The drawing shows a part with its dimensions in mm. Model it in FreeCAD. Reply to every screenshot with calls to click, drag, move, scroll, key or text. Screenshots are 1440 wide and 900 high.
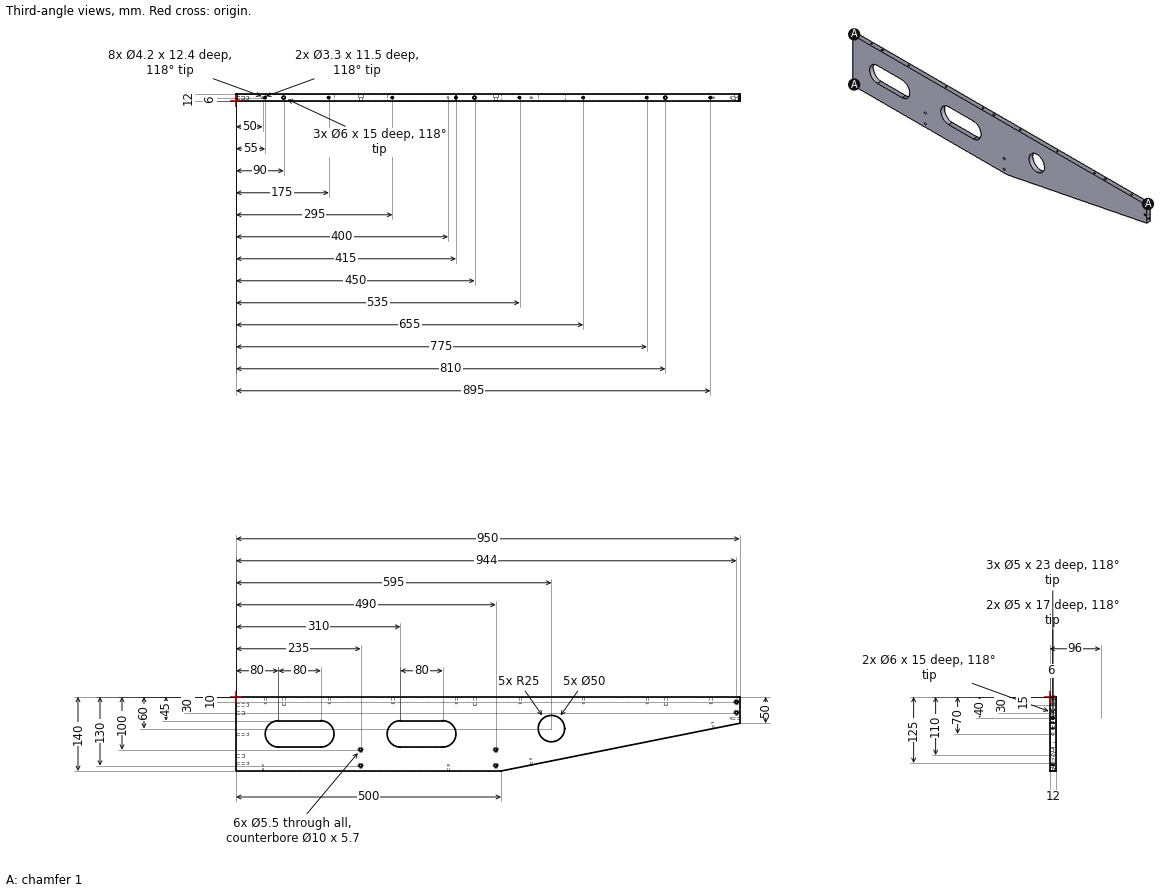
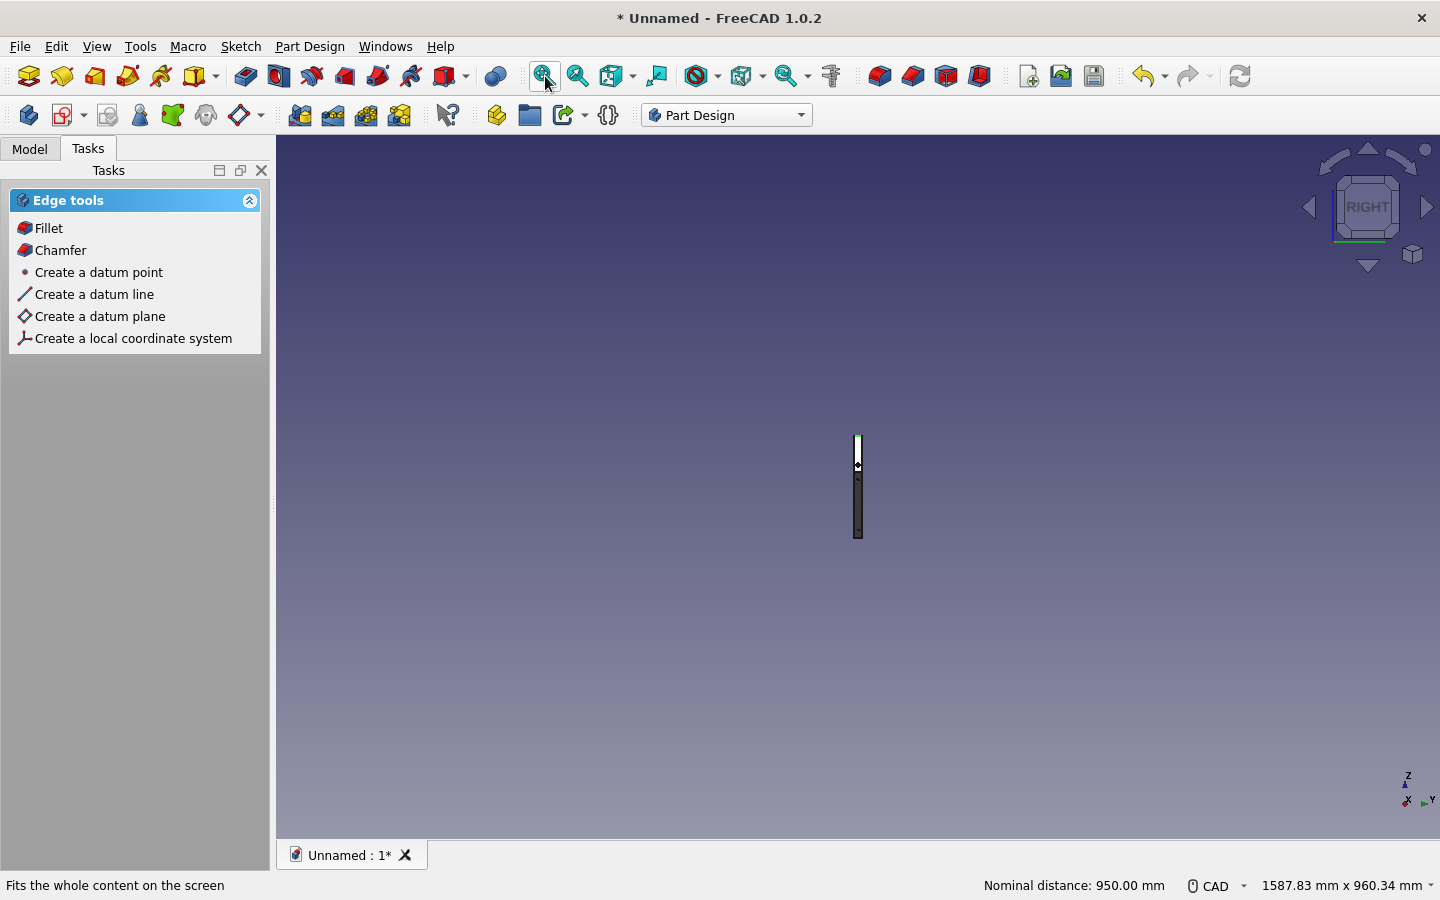
scroll(858, 537, up, 8)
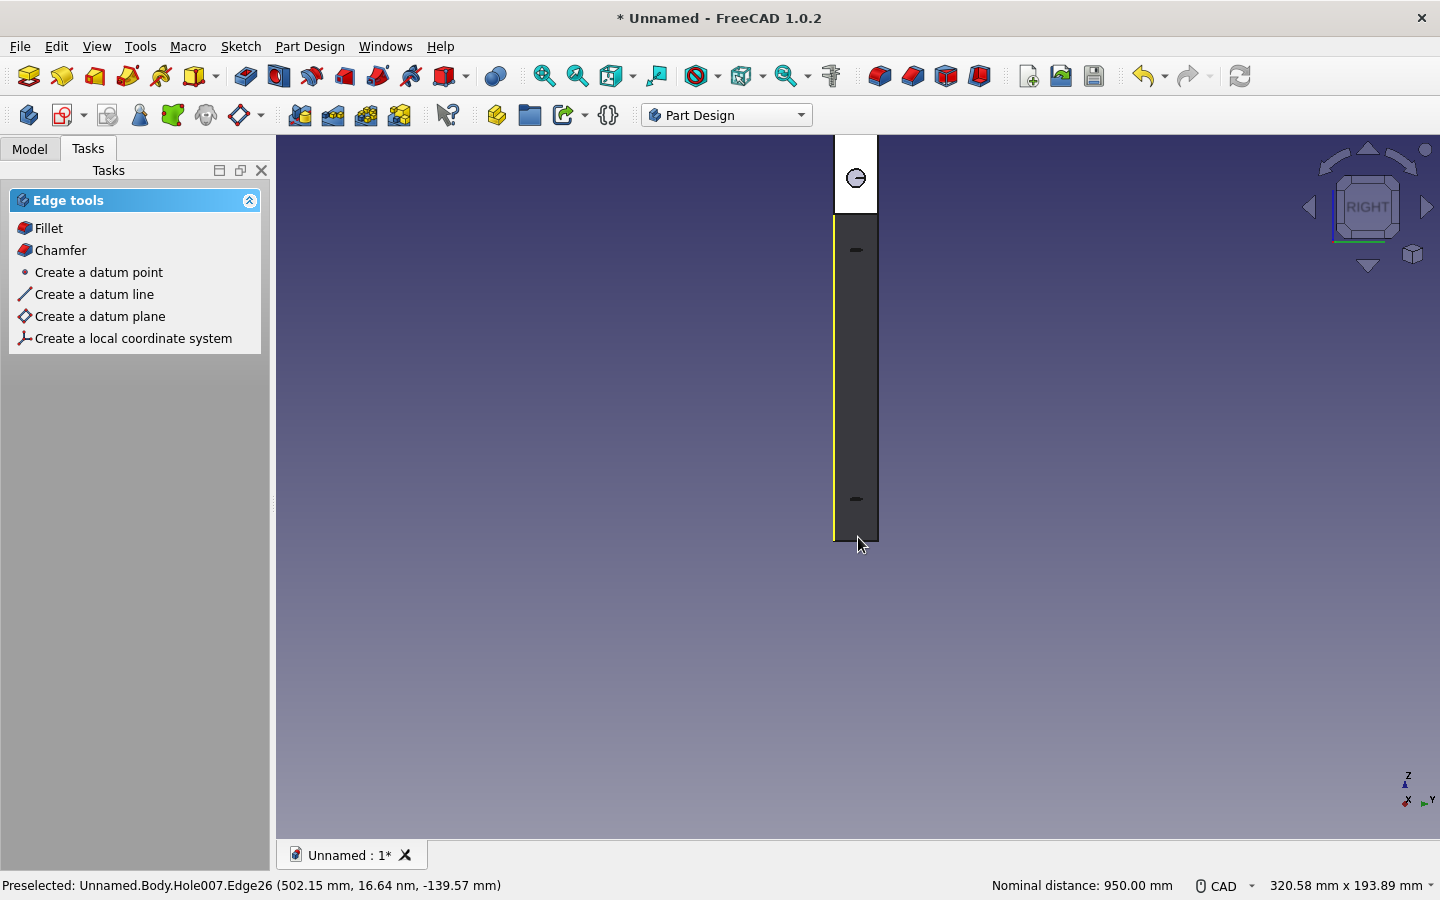
click(545, 76)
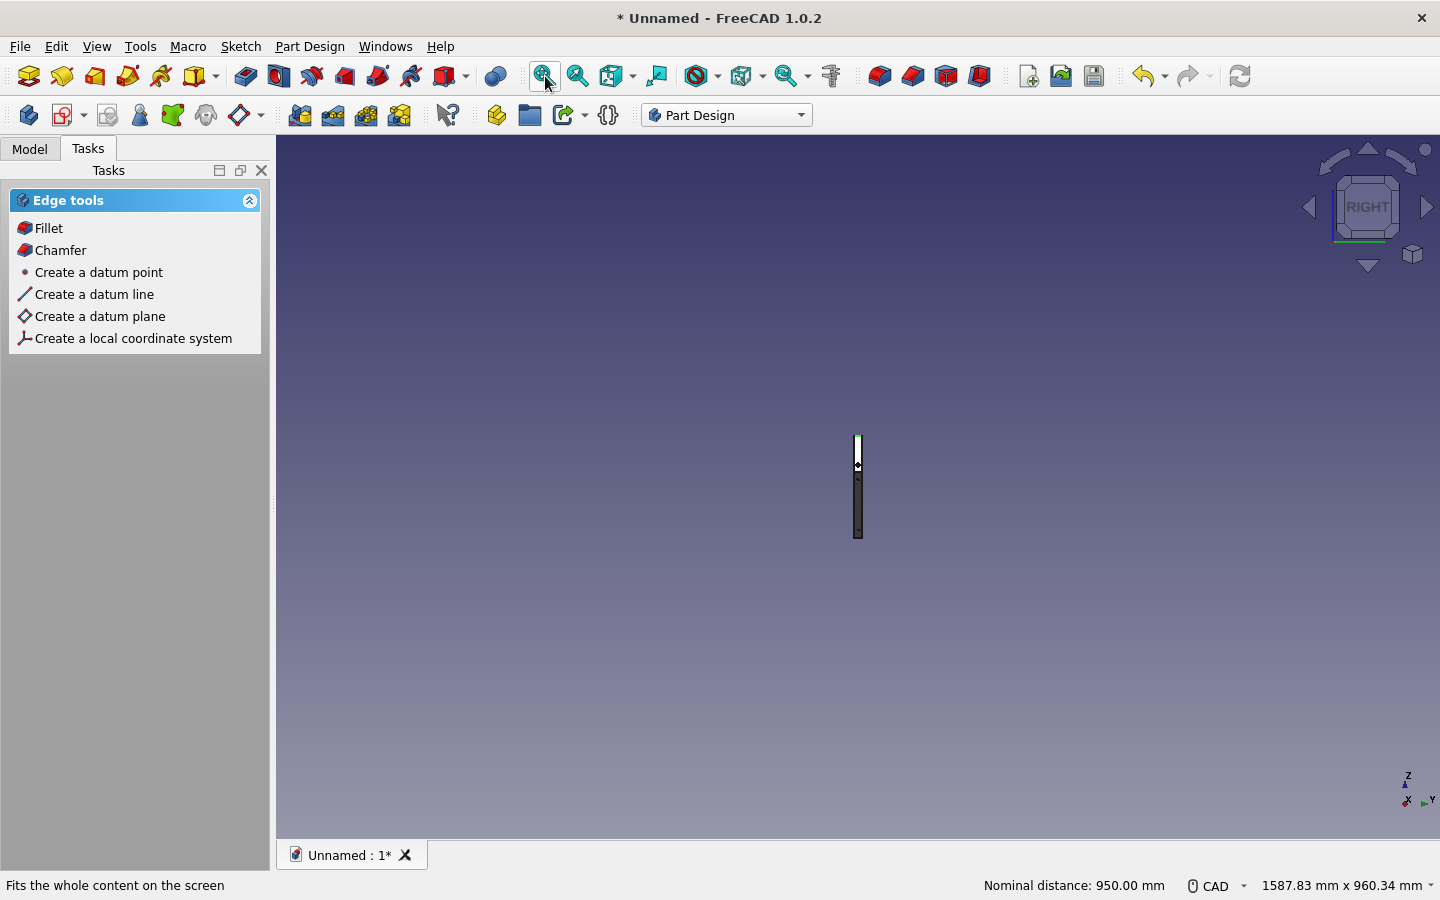
key(5)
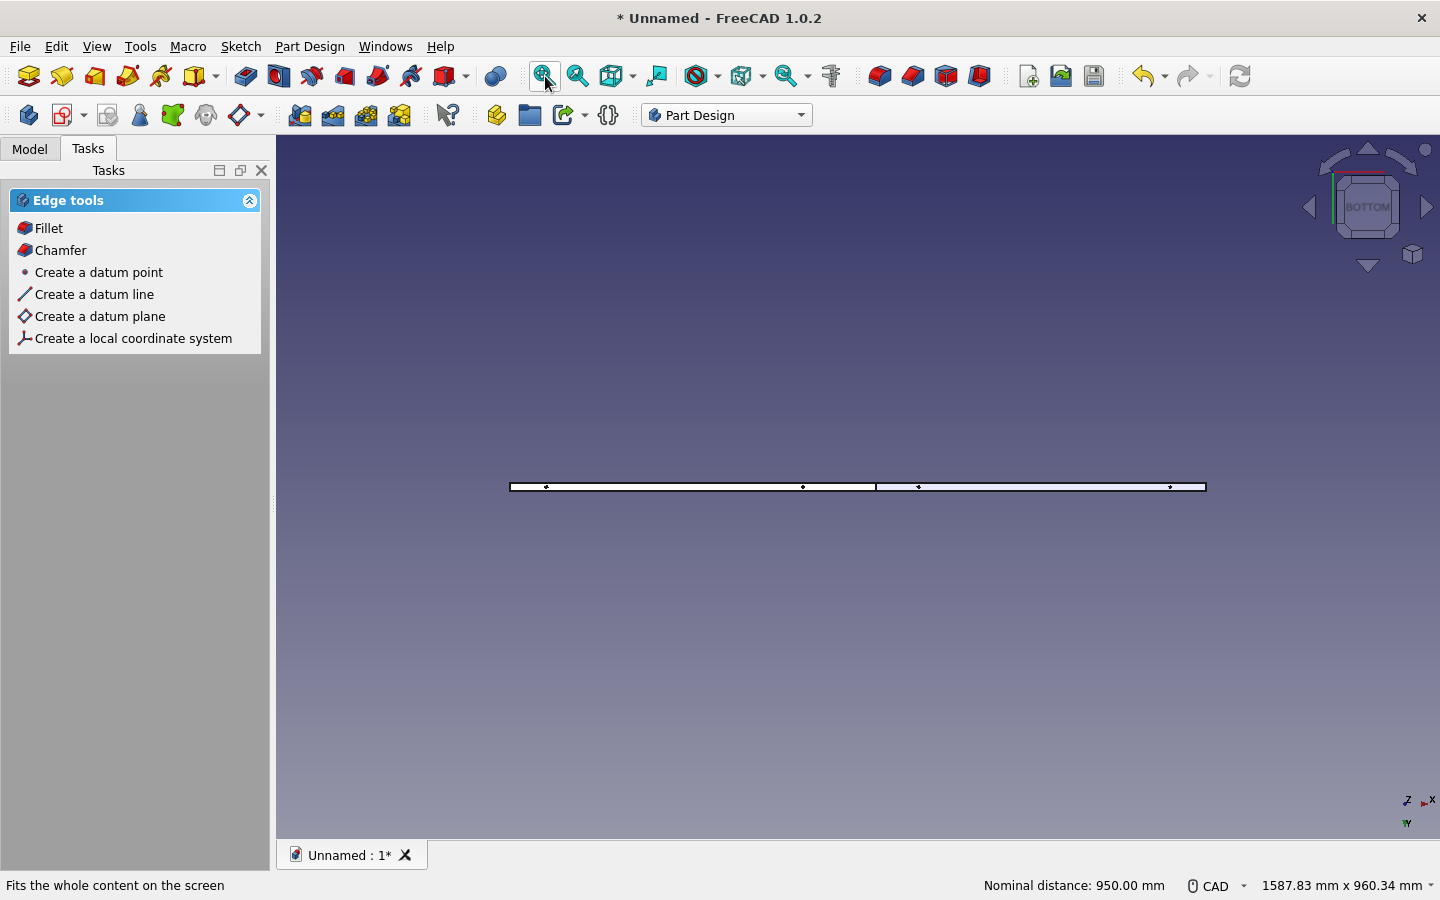
click(510, 488, ctrl)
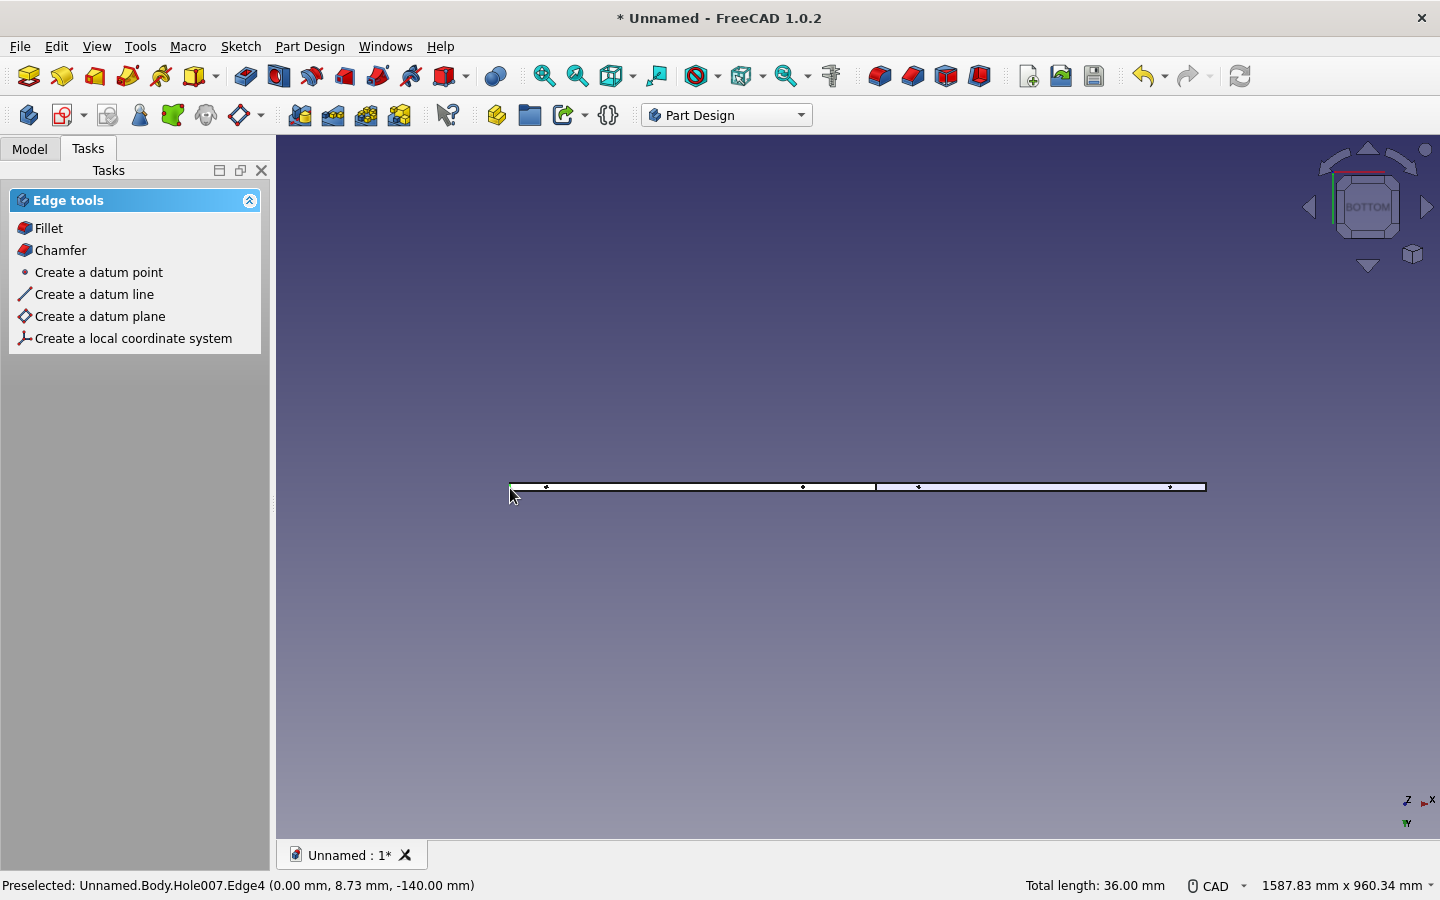
click(913, 76)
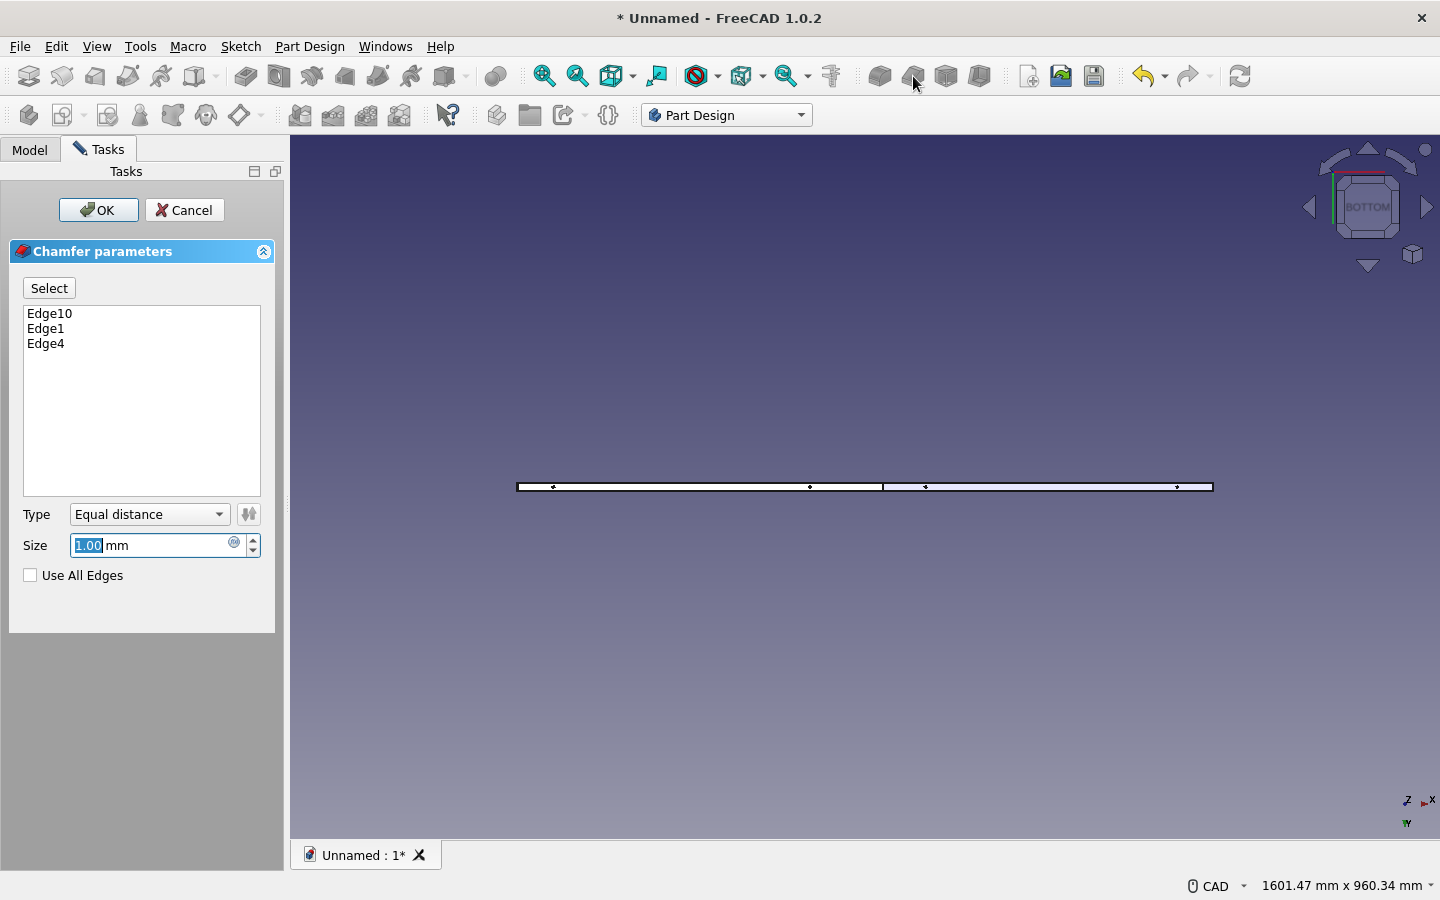
text(1)
key(Tab)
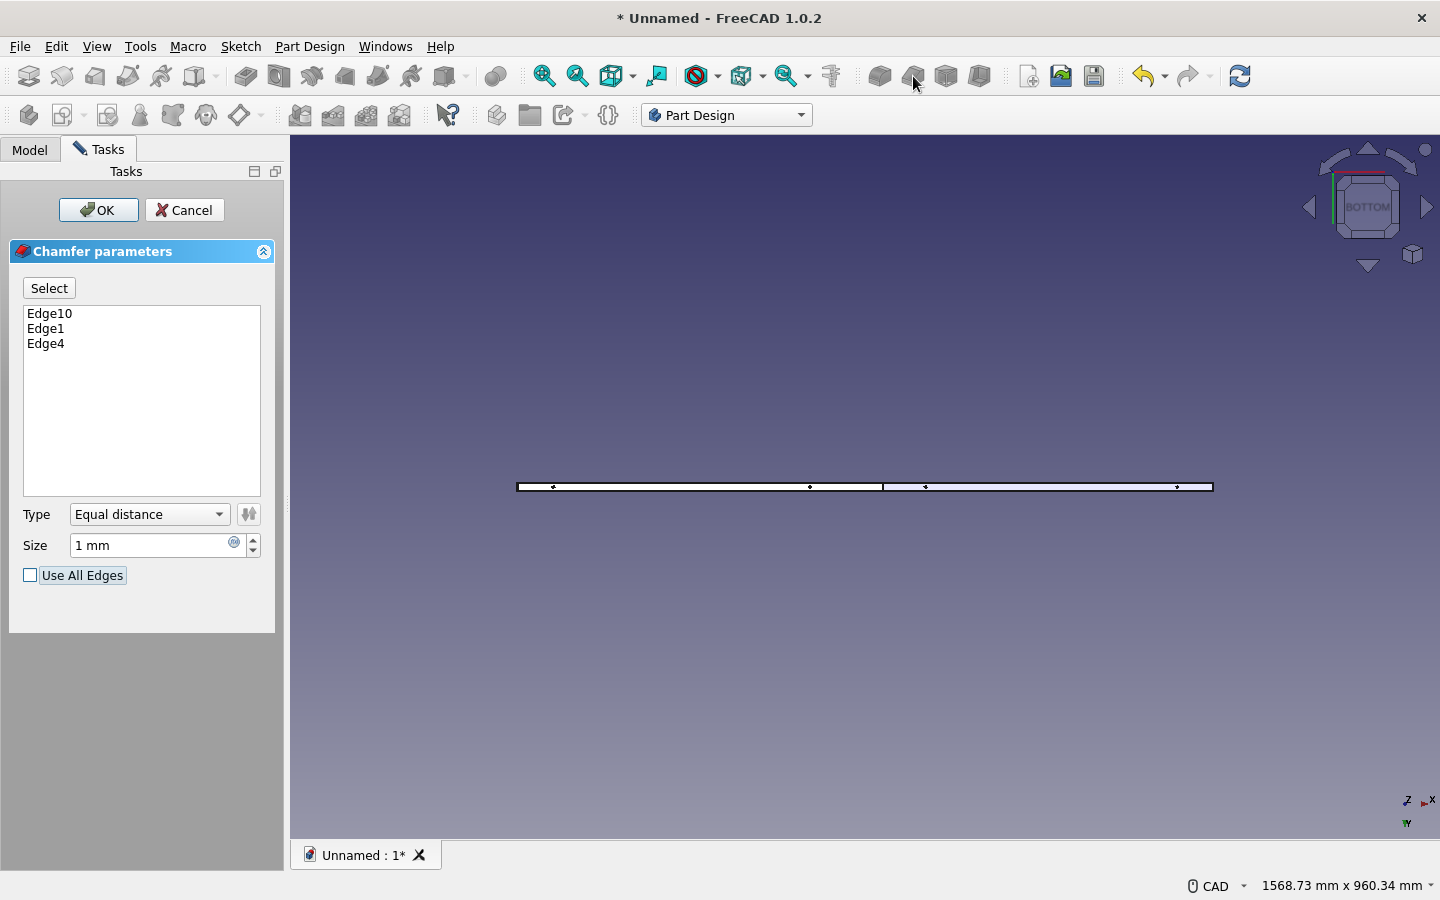
click(99, 210)